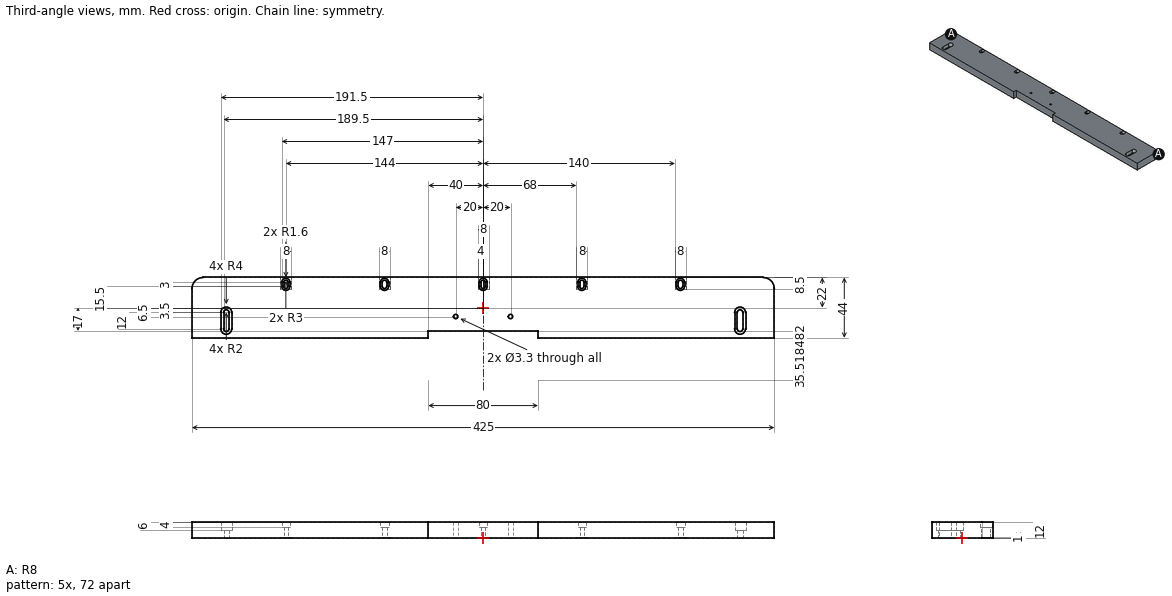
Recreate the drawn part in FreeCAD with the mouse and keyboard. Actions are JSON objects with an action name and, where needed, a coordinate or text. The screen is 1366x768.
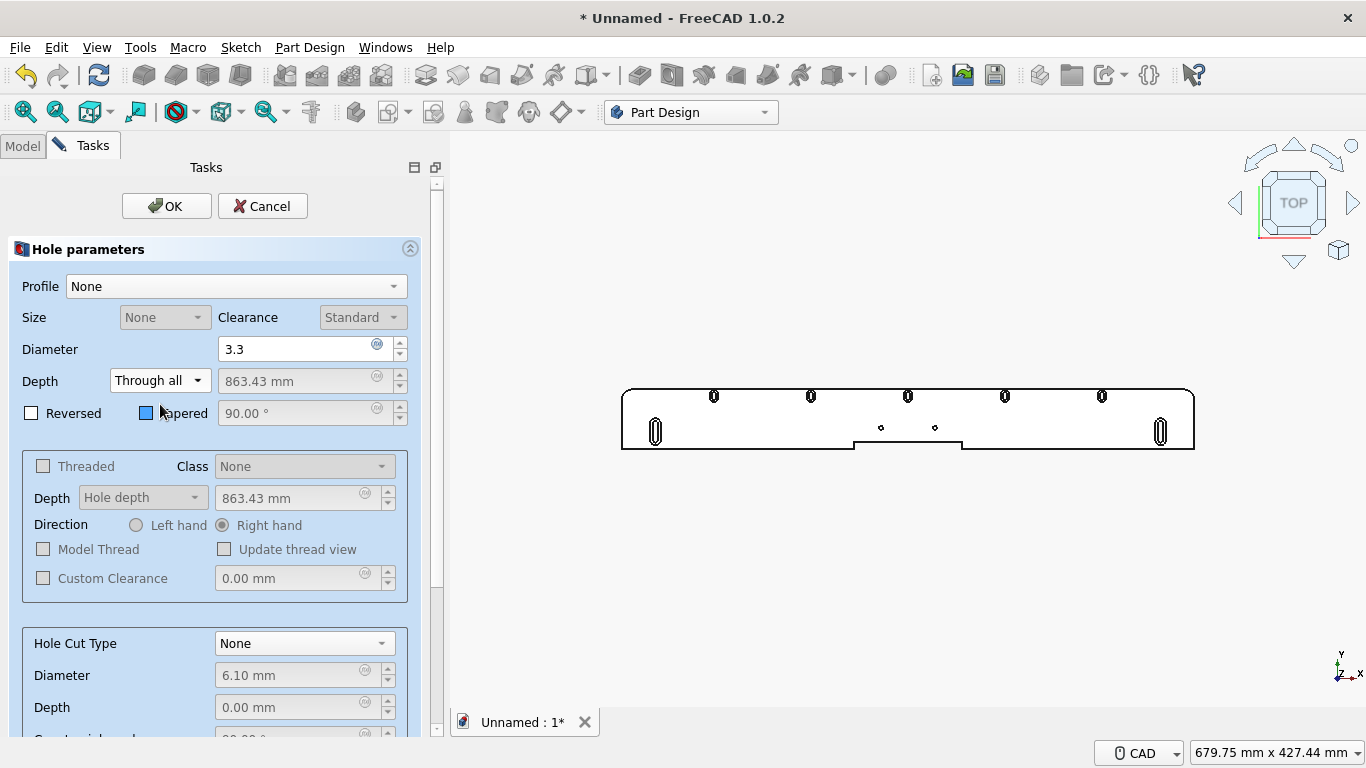
{"action": "left_click", "coordinate": [167, 206]}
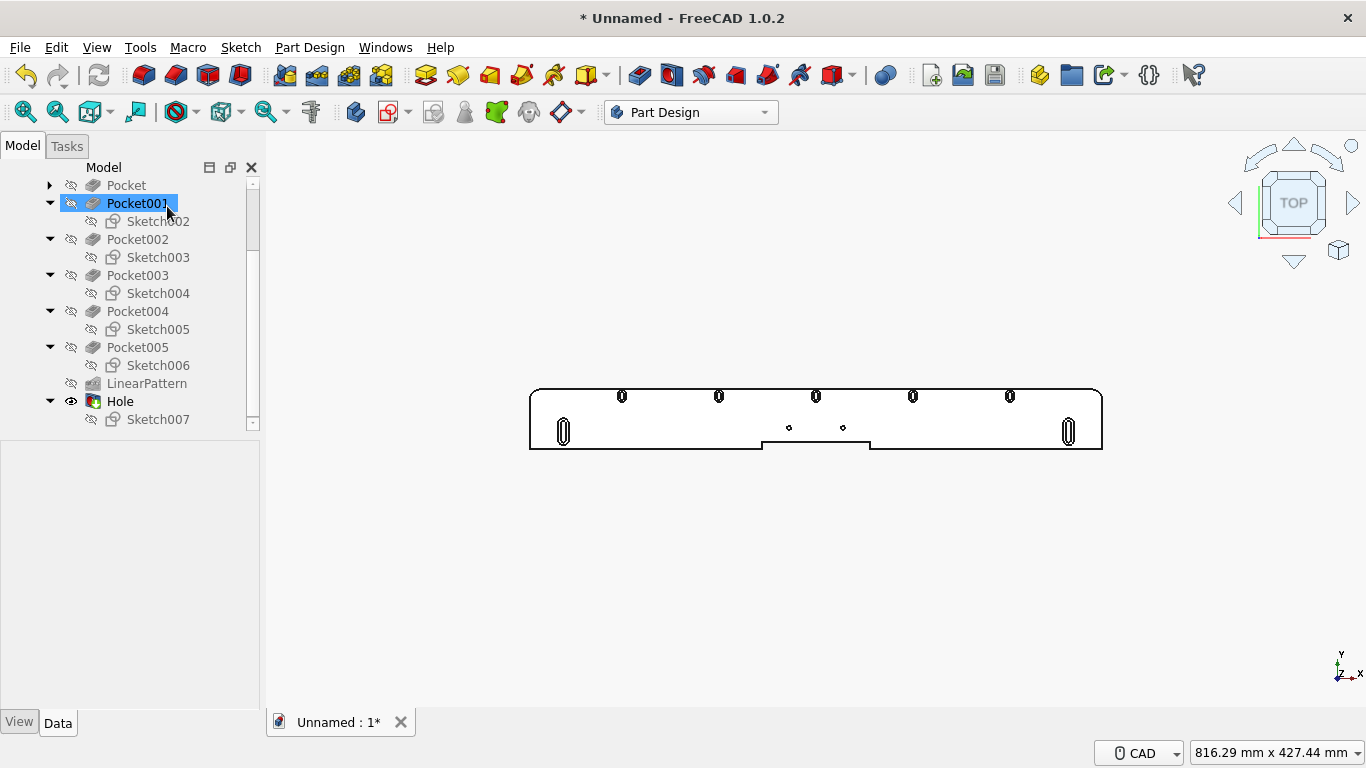
{"action": "key", "text": "0"}